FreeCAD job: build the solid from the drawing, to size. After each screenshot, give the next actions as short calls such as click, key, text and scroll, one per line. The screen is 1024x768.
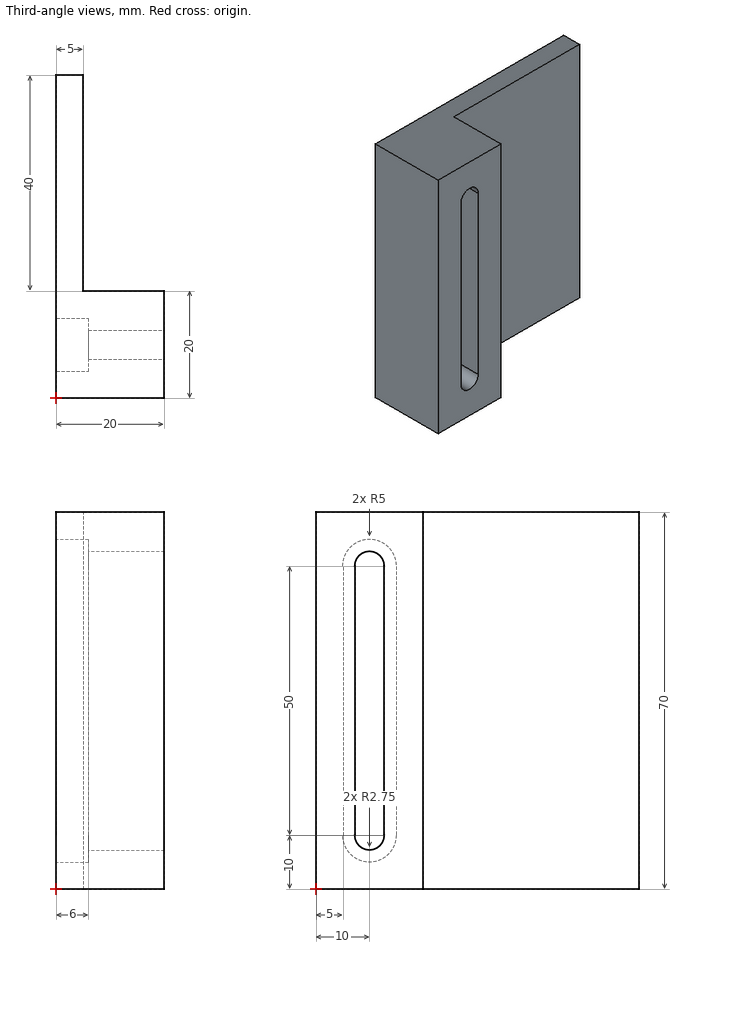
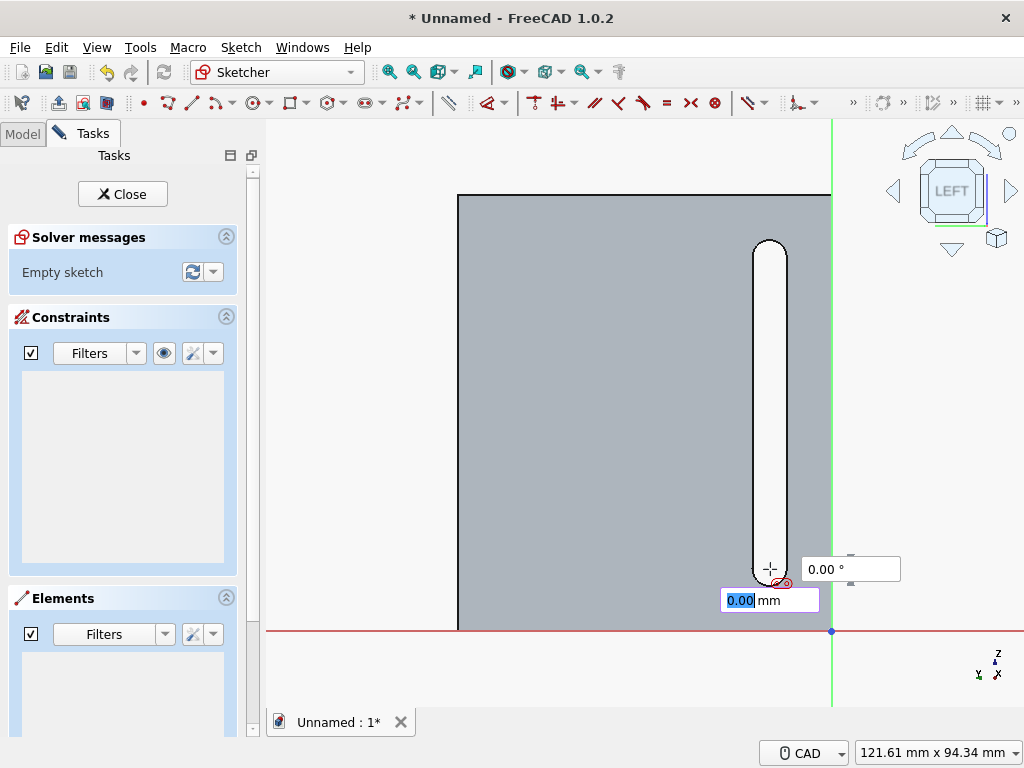
click(770, 257)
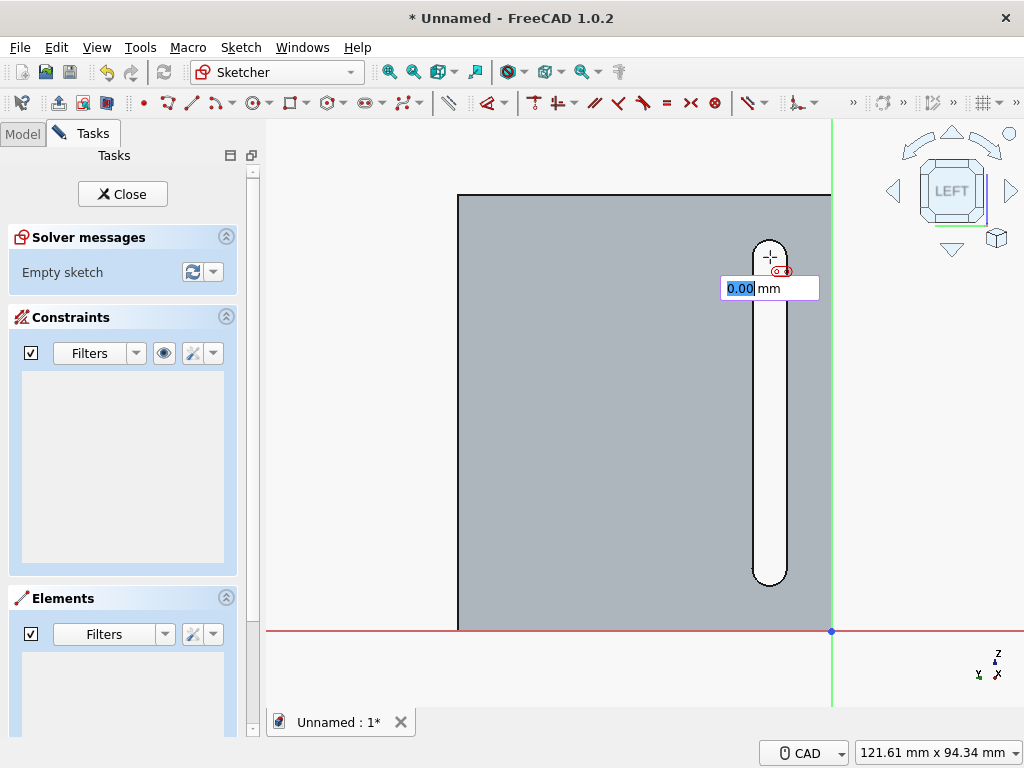
click(801, 413)
key(Escape)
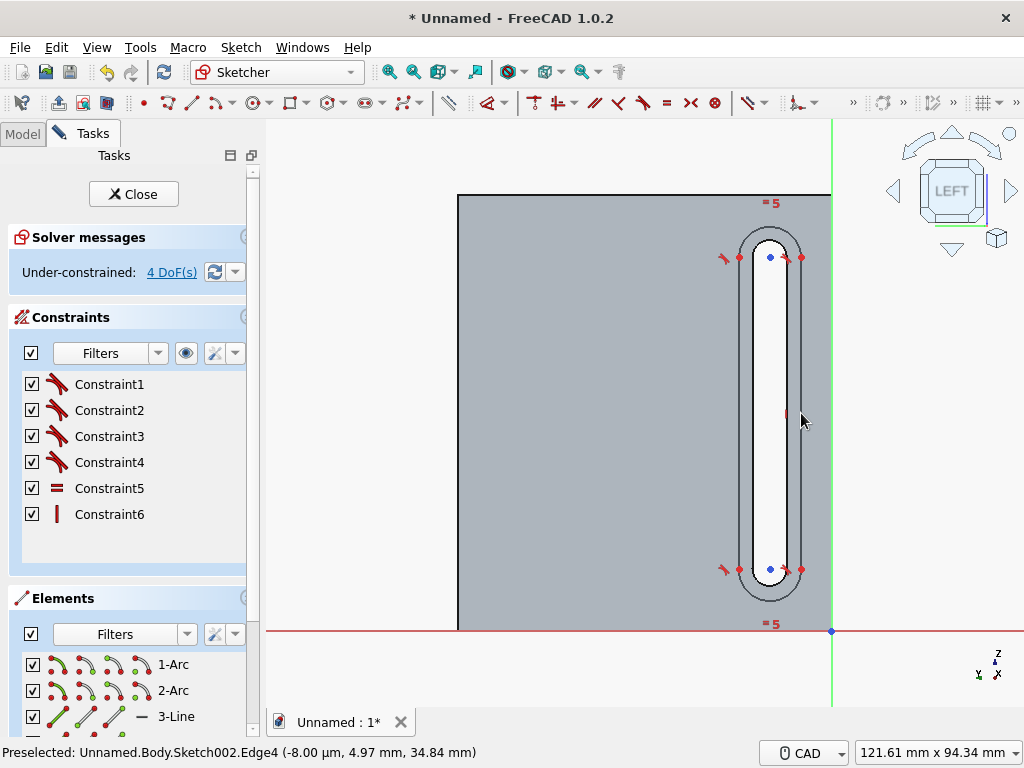
click(488, 104)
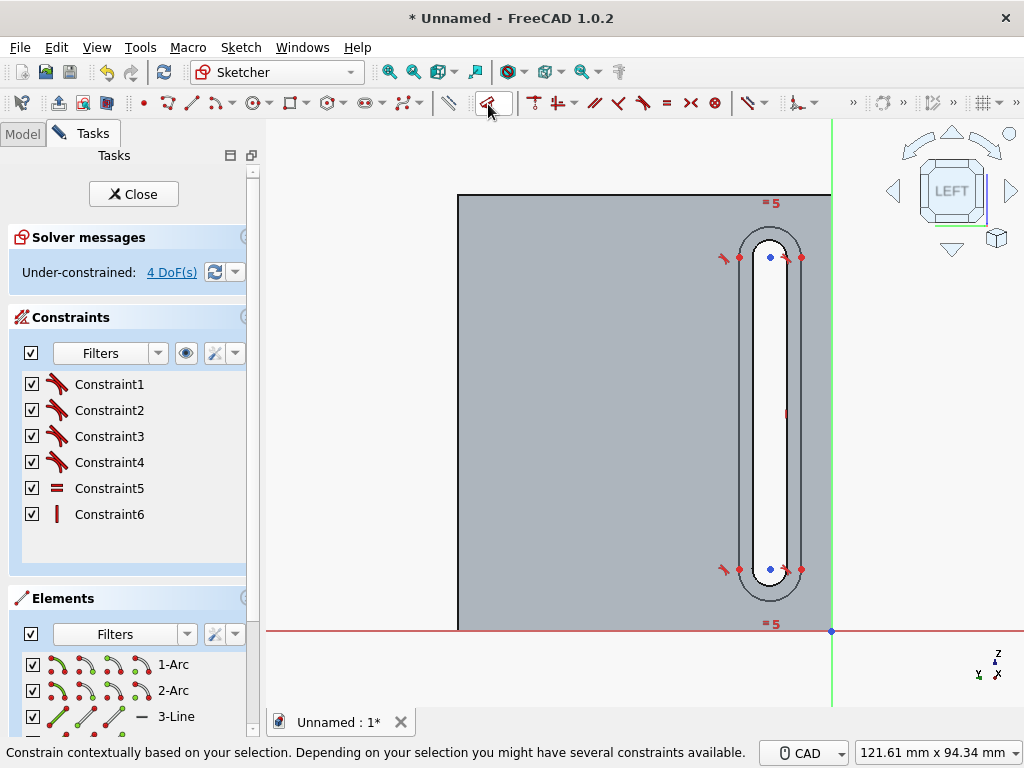
scroll(752, 595, up, 2)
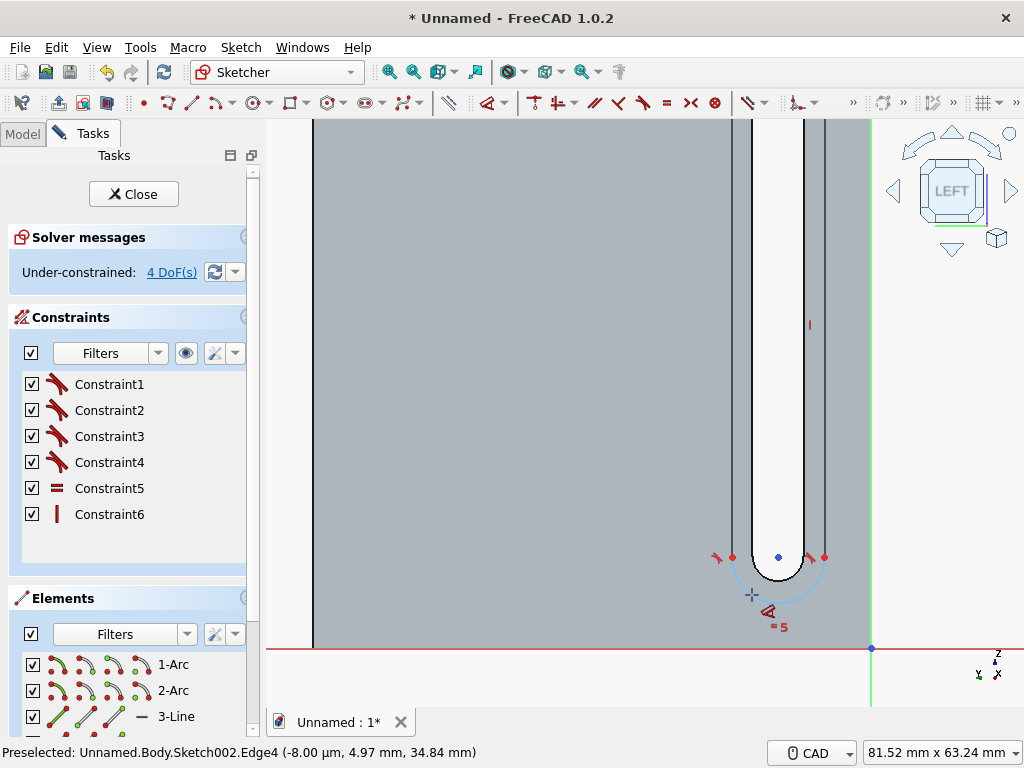
click(751, 595)
click(732, 621)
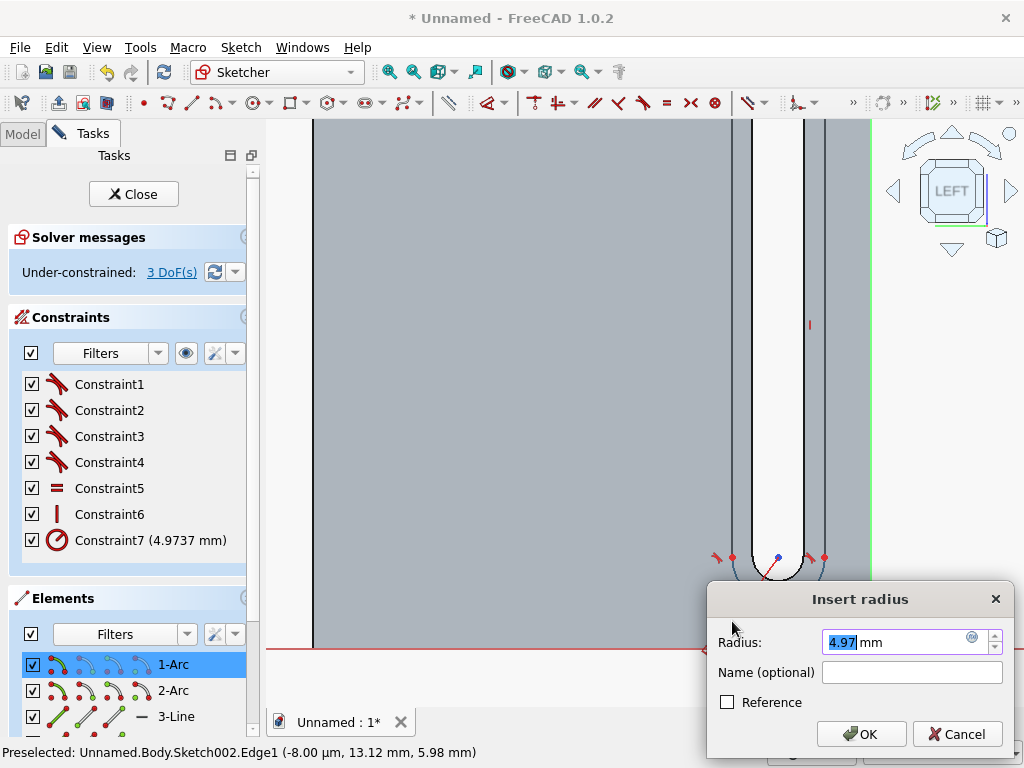
text(5)
key(Return)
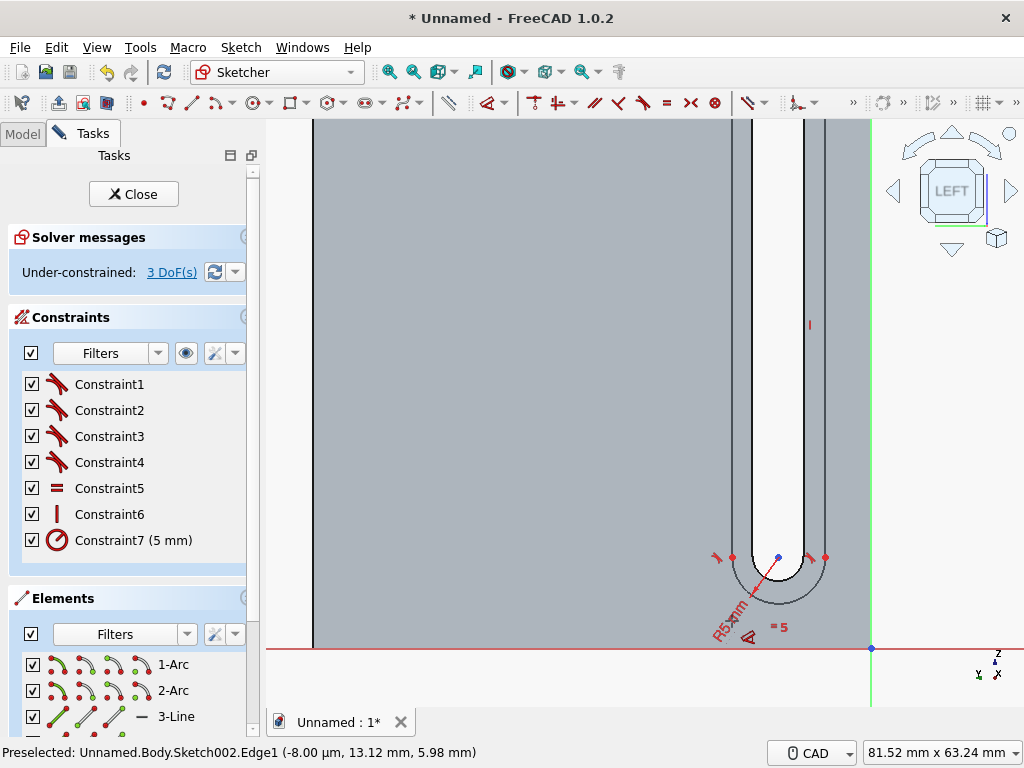
click(732, 418)
click(698, 352)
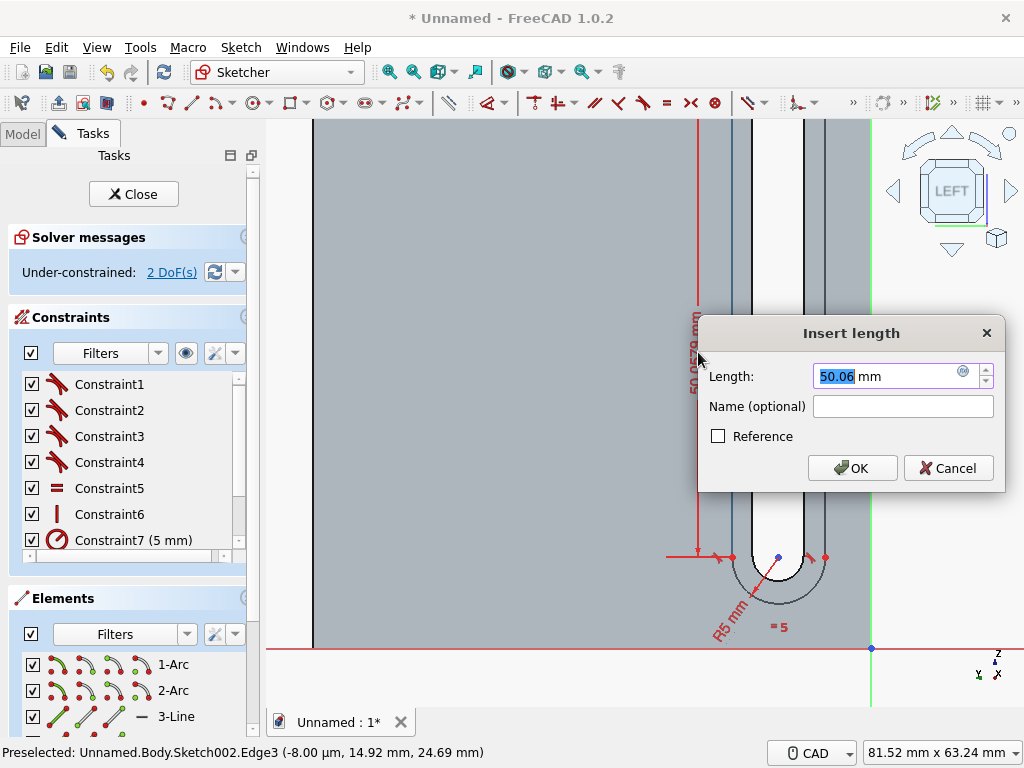
text(50)
key(Return)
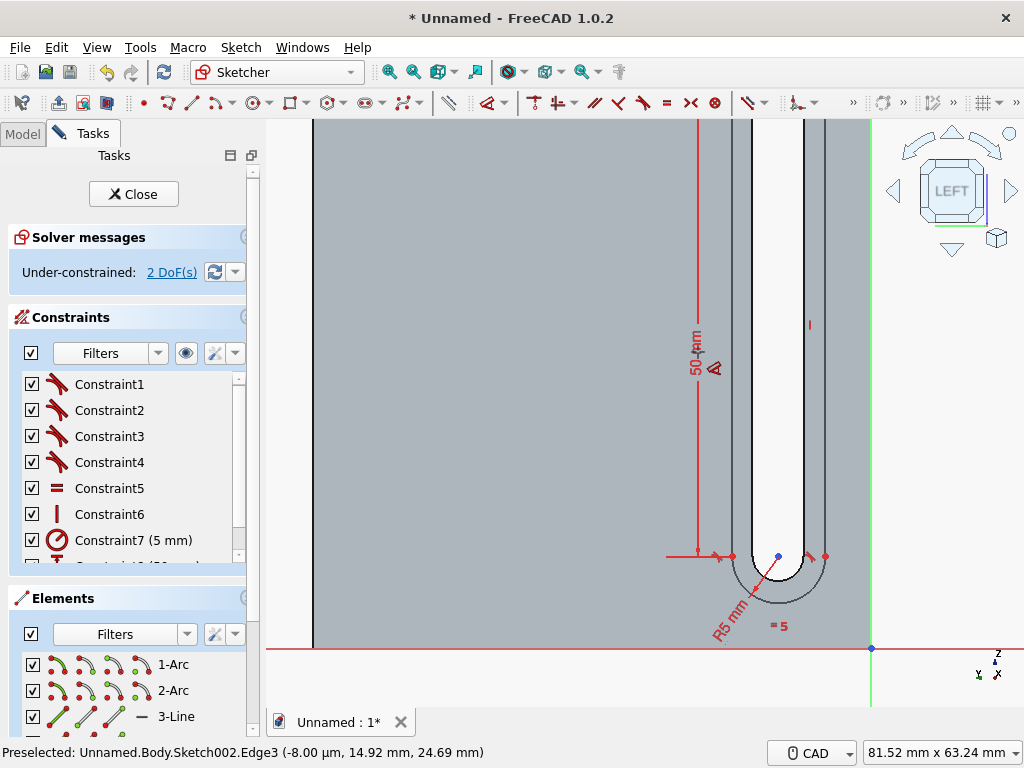
click(825, 557)
click(842, 523)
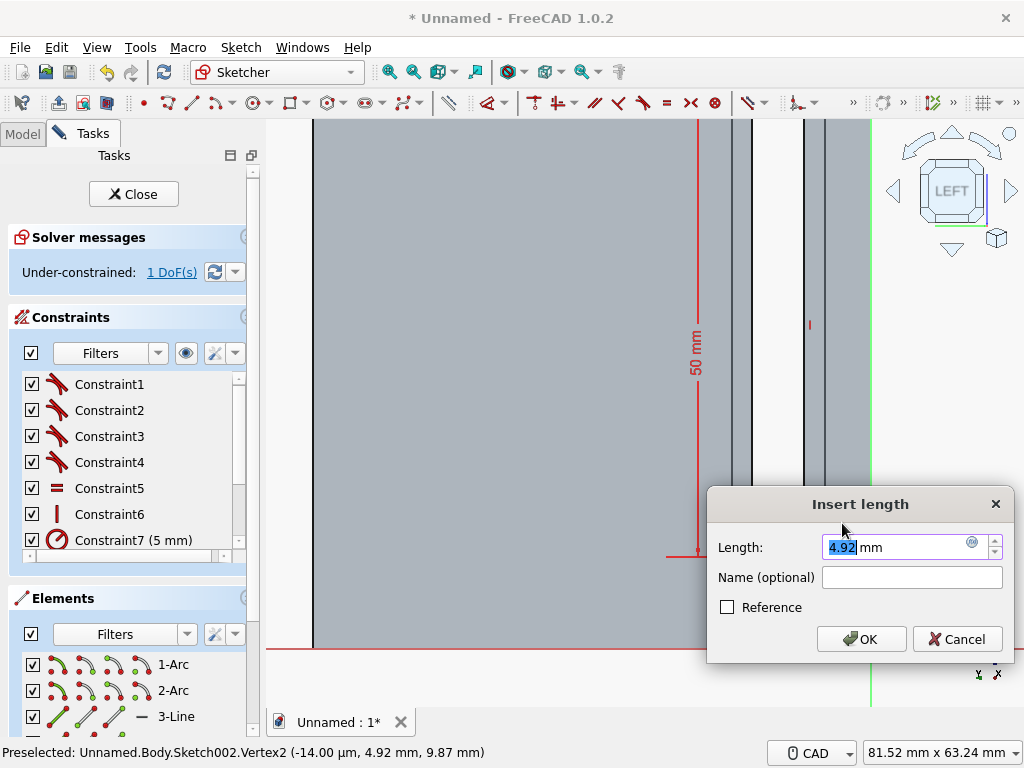
text(5)
key(Return)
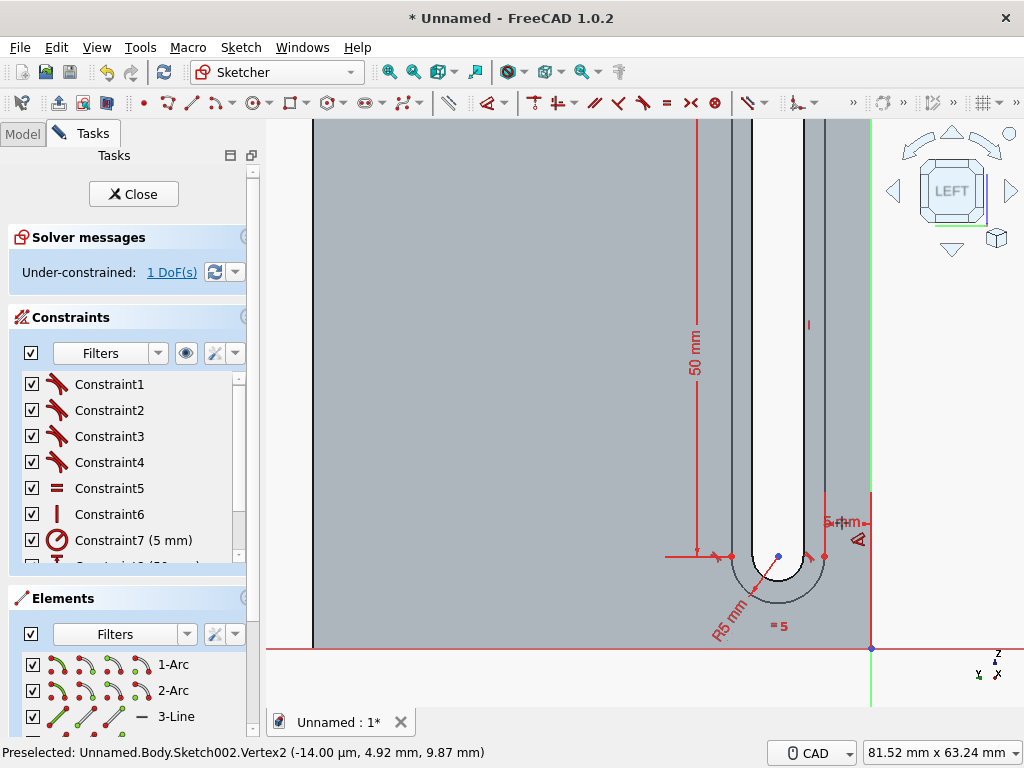
click(732, 557)
click(698, 582)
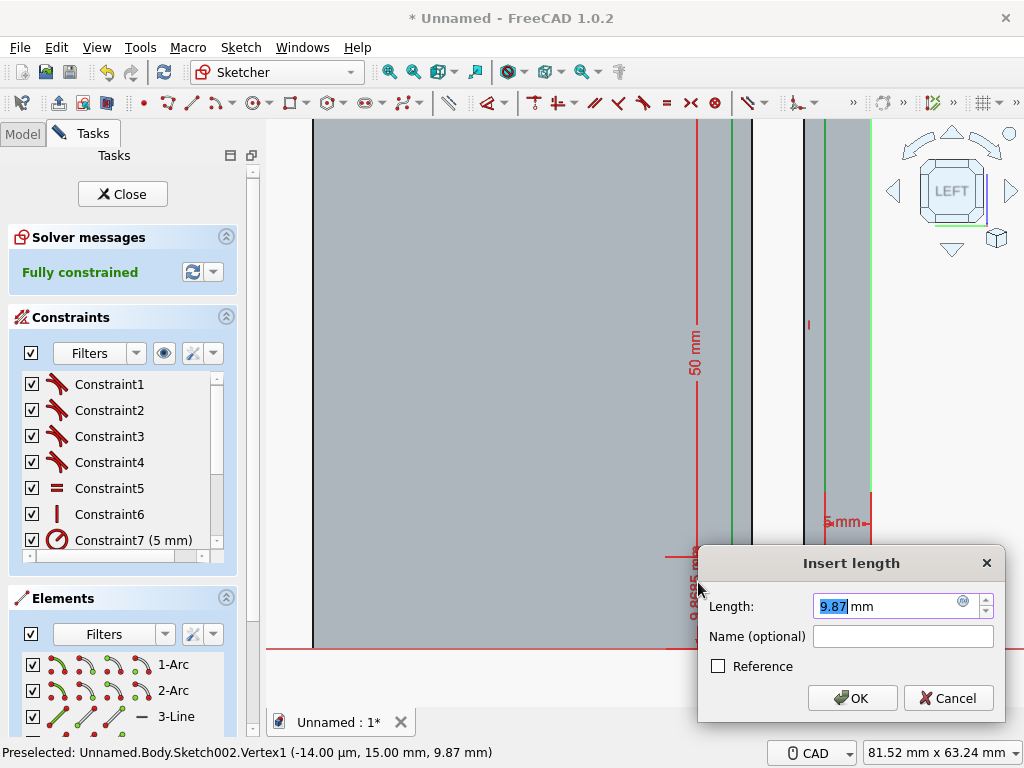
text(10)
key(Return)
key(Escape)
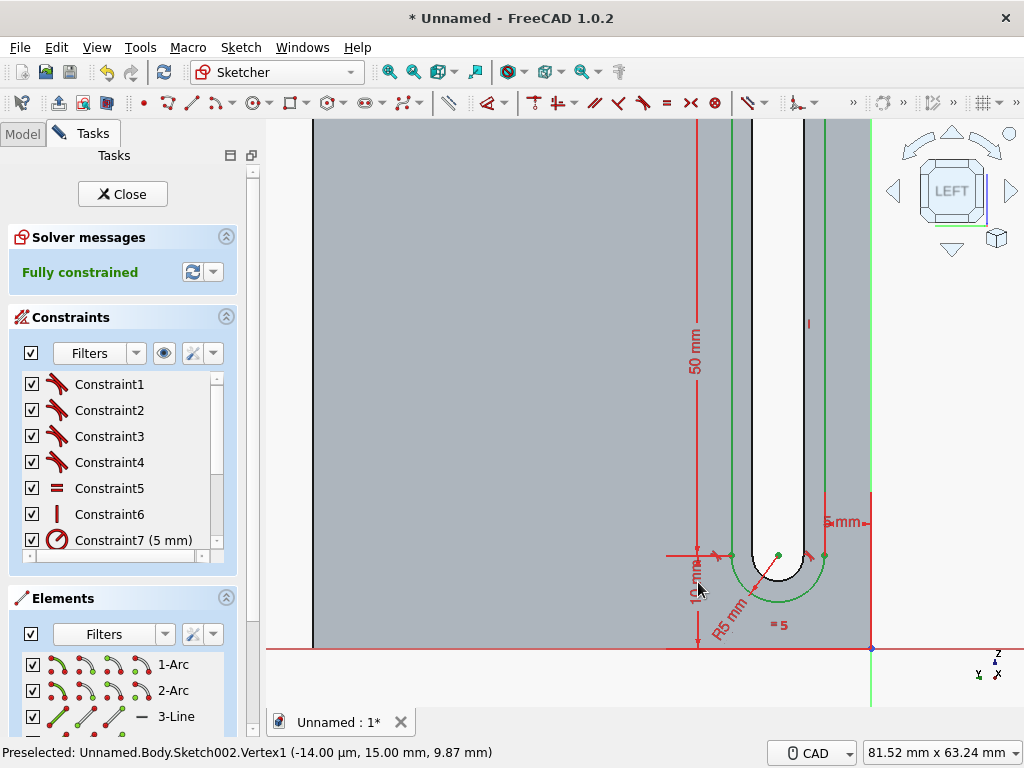
click(123, 194)